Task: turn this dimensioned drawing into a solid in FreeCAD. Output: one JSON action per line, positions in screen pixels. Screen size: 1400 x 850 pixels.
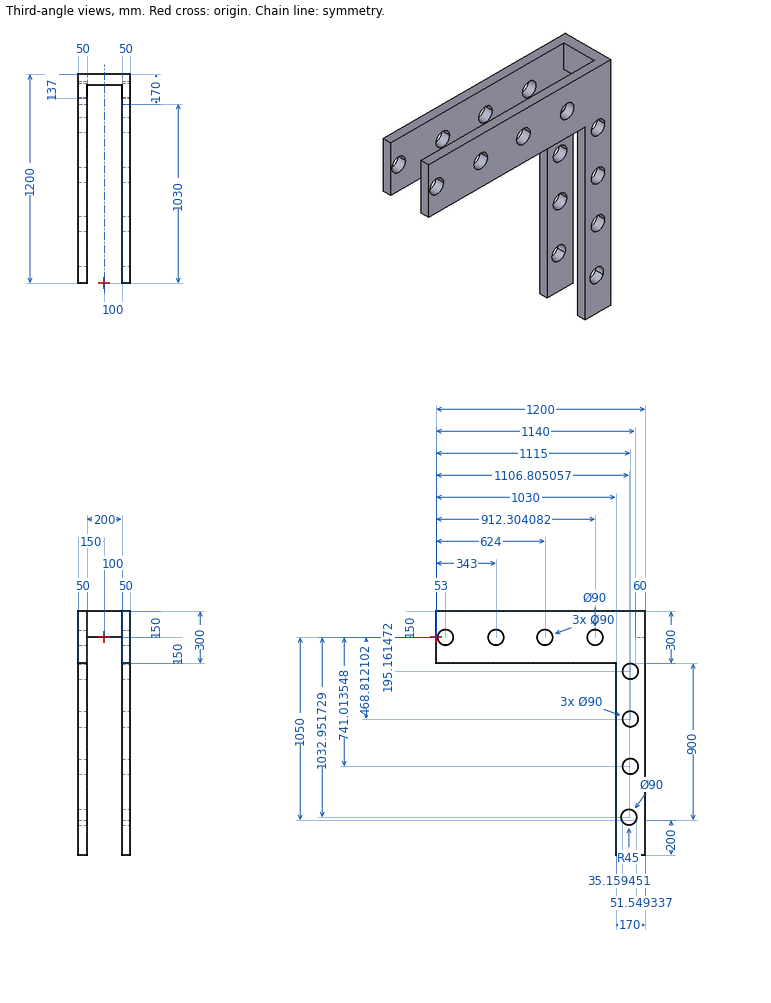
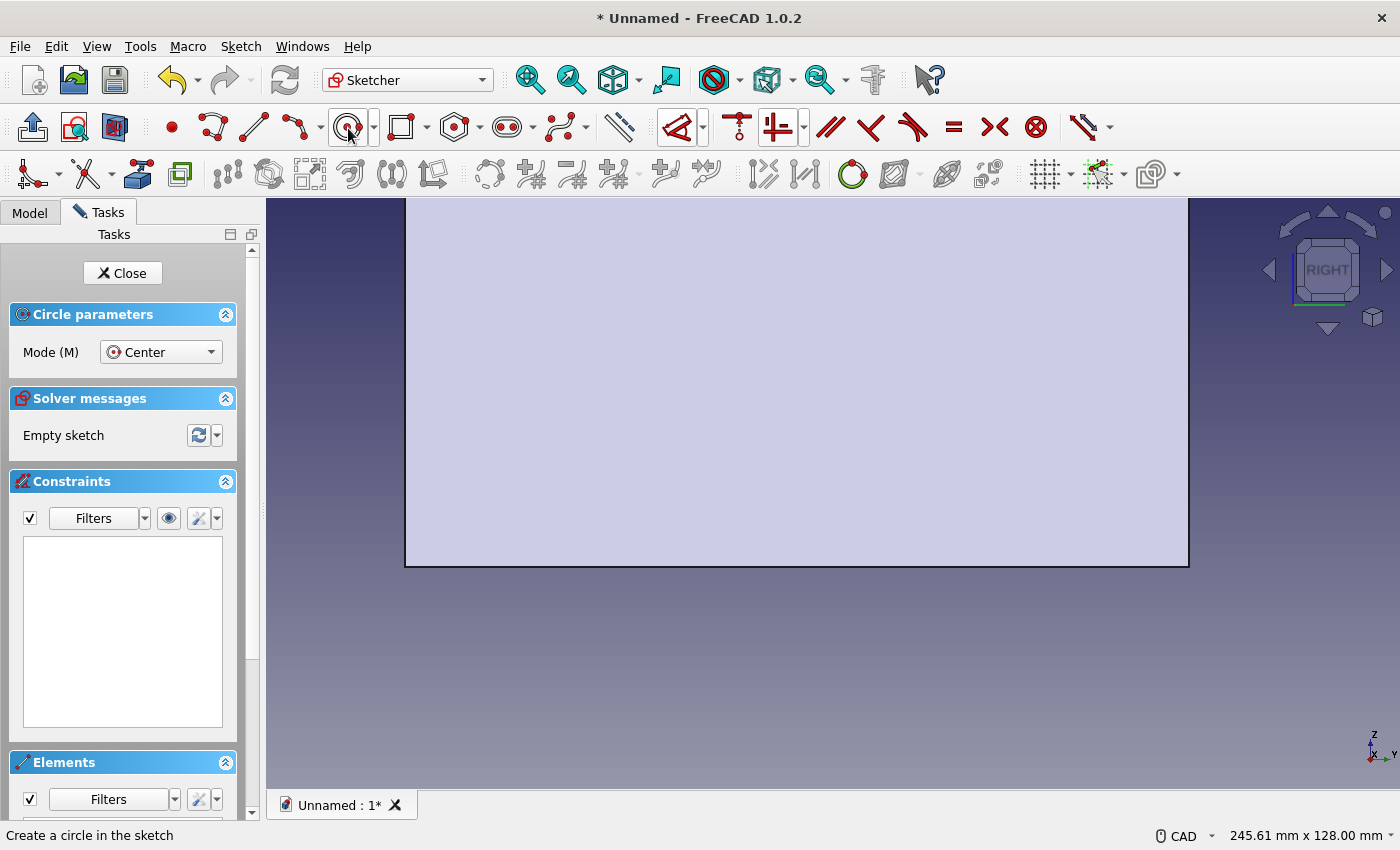
{"action": "left_click", "coordinate": [759, 488]}
{"action": "left_click", "coordinate": [906, 341]}
{"action": "key", "text": "Escape"}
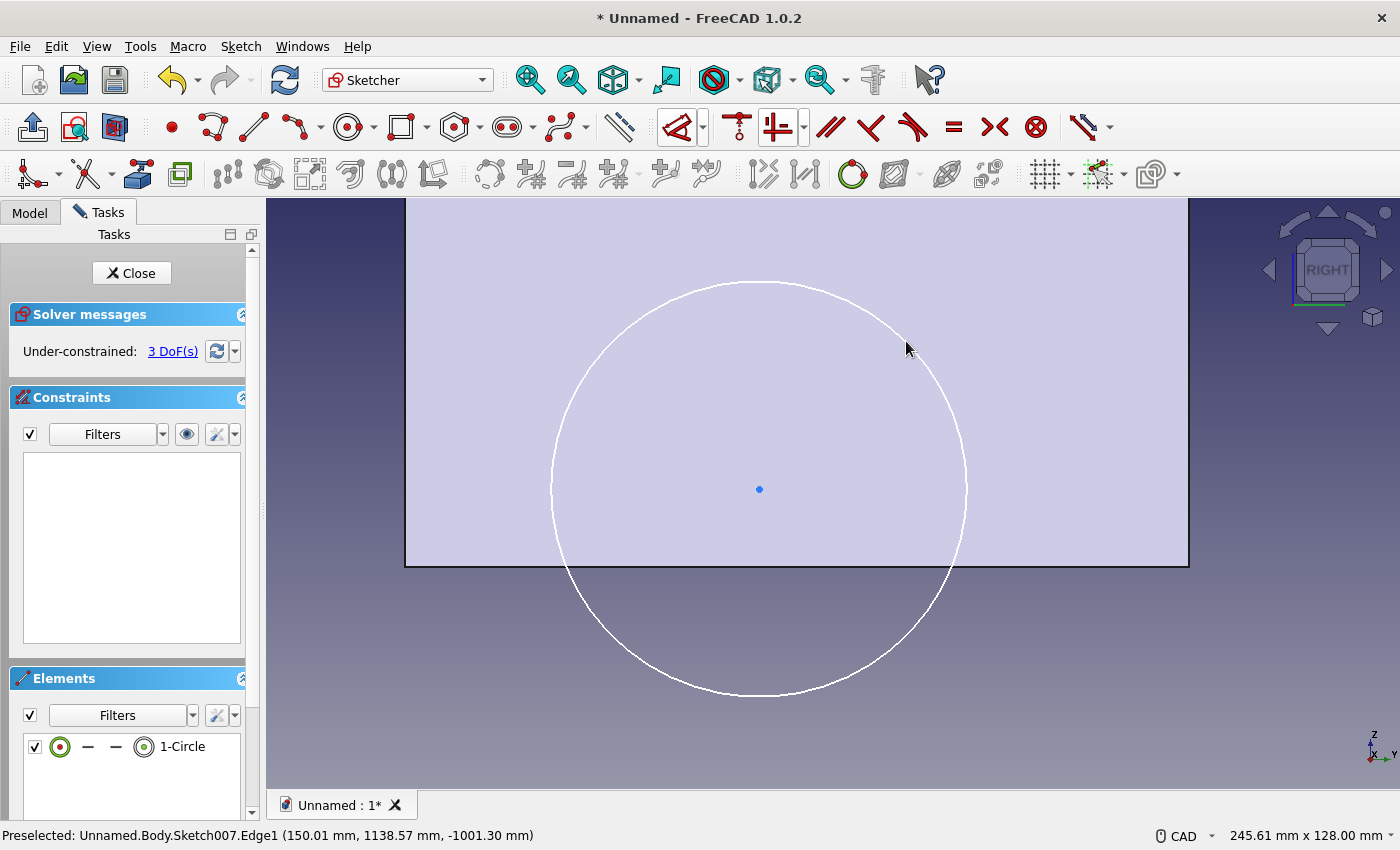
{"action": "left_click", "coordinate": [906, 342]}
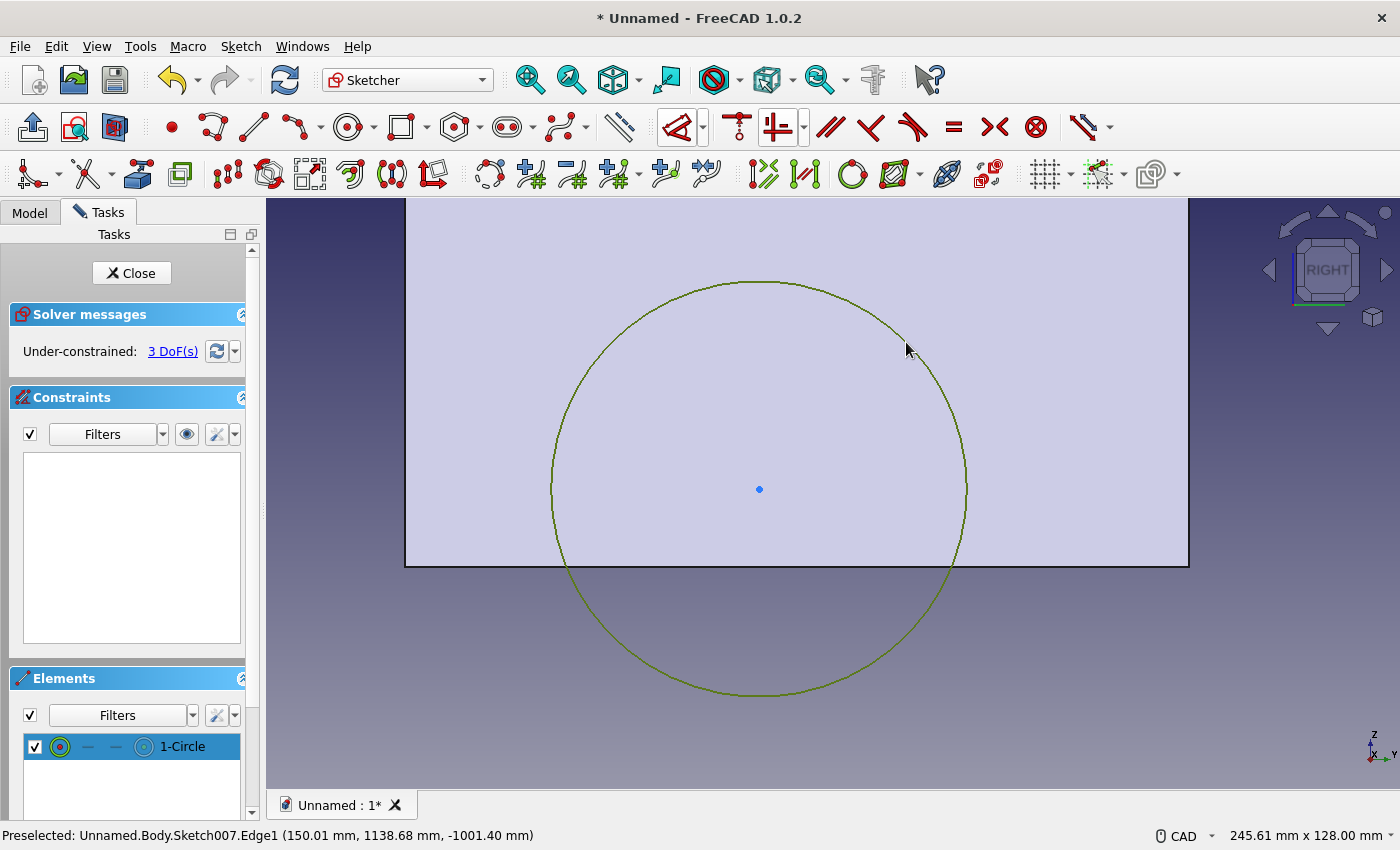
{"action": "key", "text": "k o"}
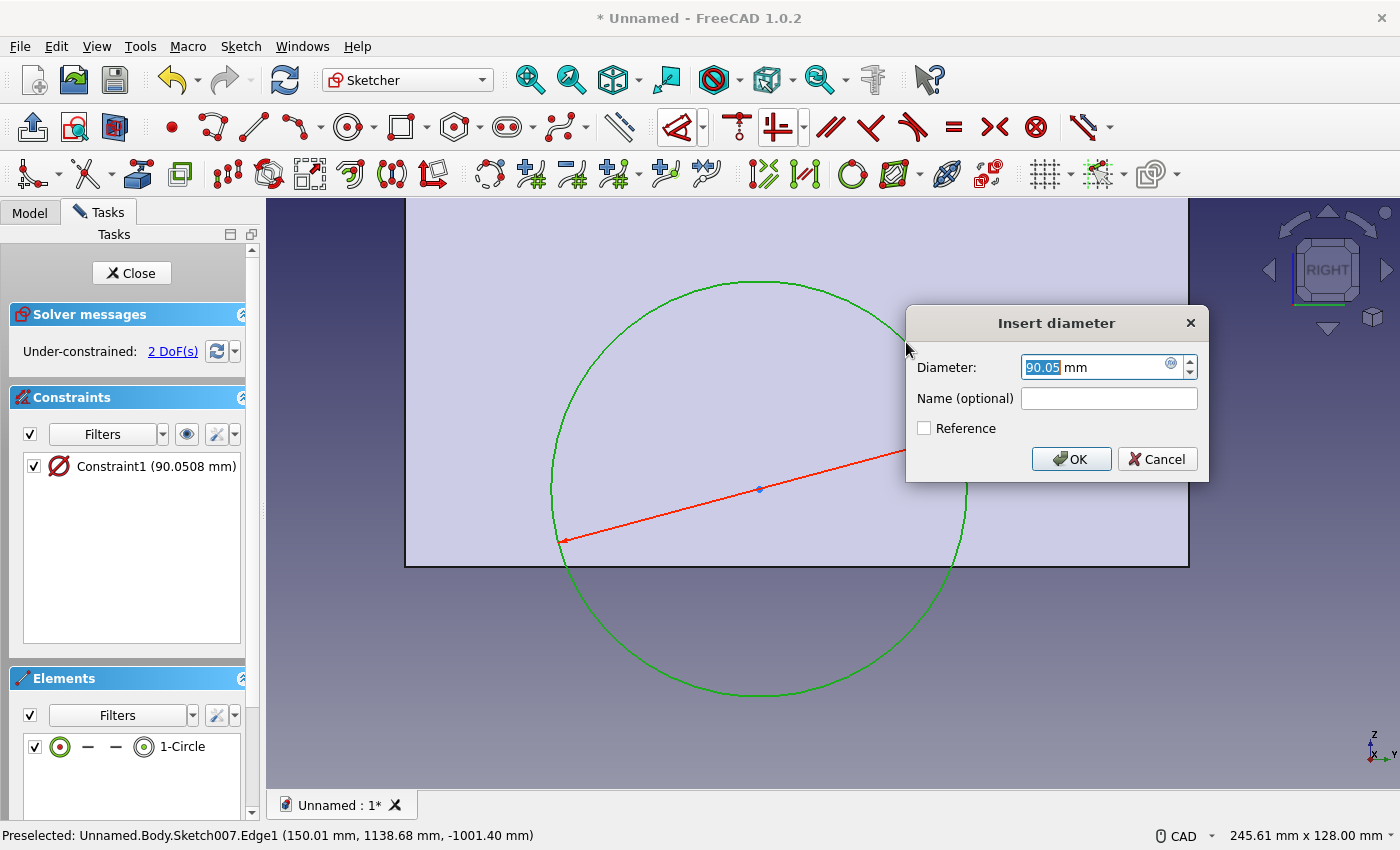
{"action": "type", "text": "90"}
{"action": "key", "text": "Return"}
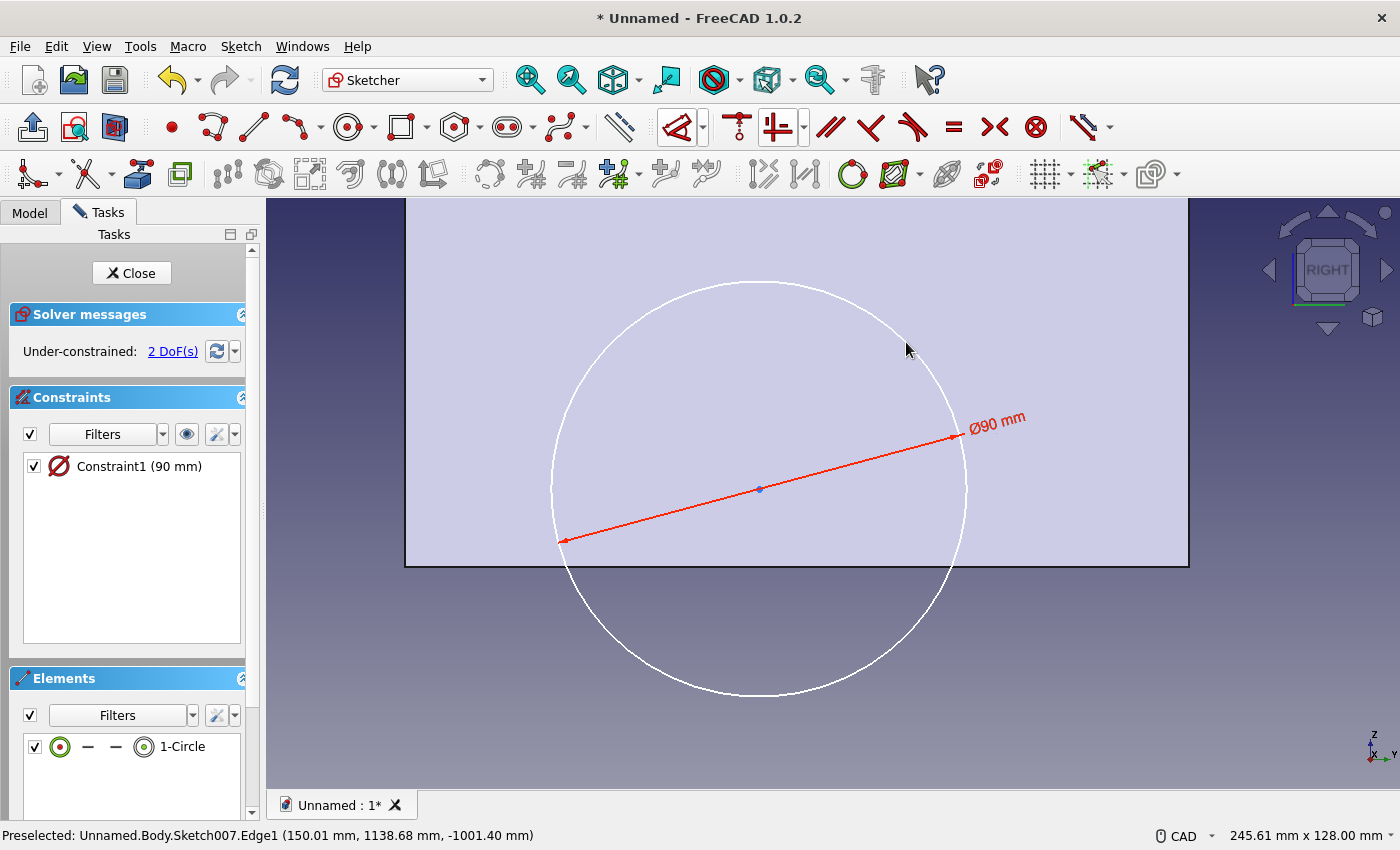
{"action": "left_click", "coordinate": [759, 489]}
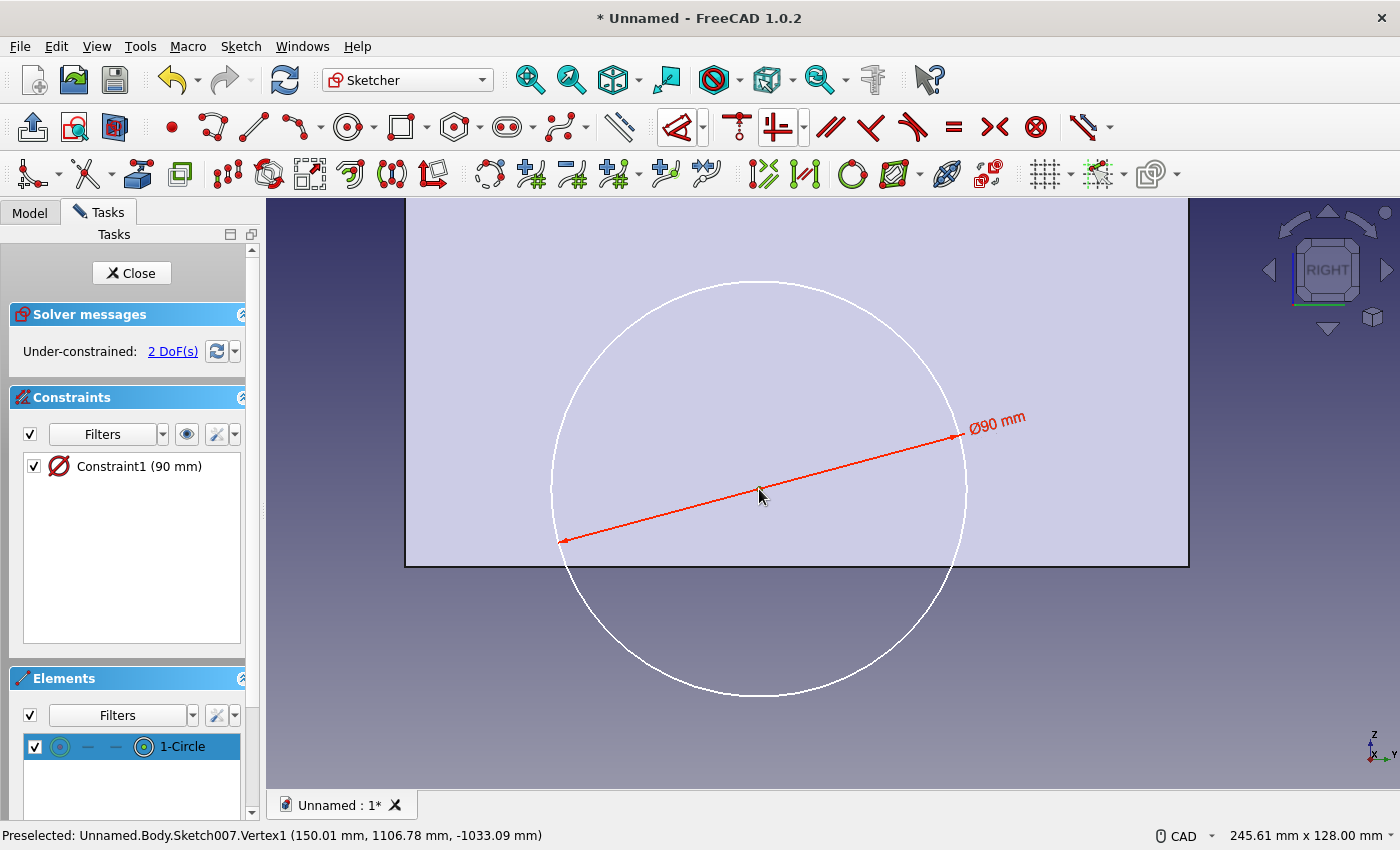
{"action": "left_click", "coordinate": [702, 128]}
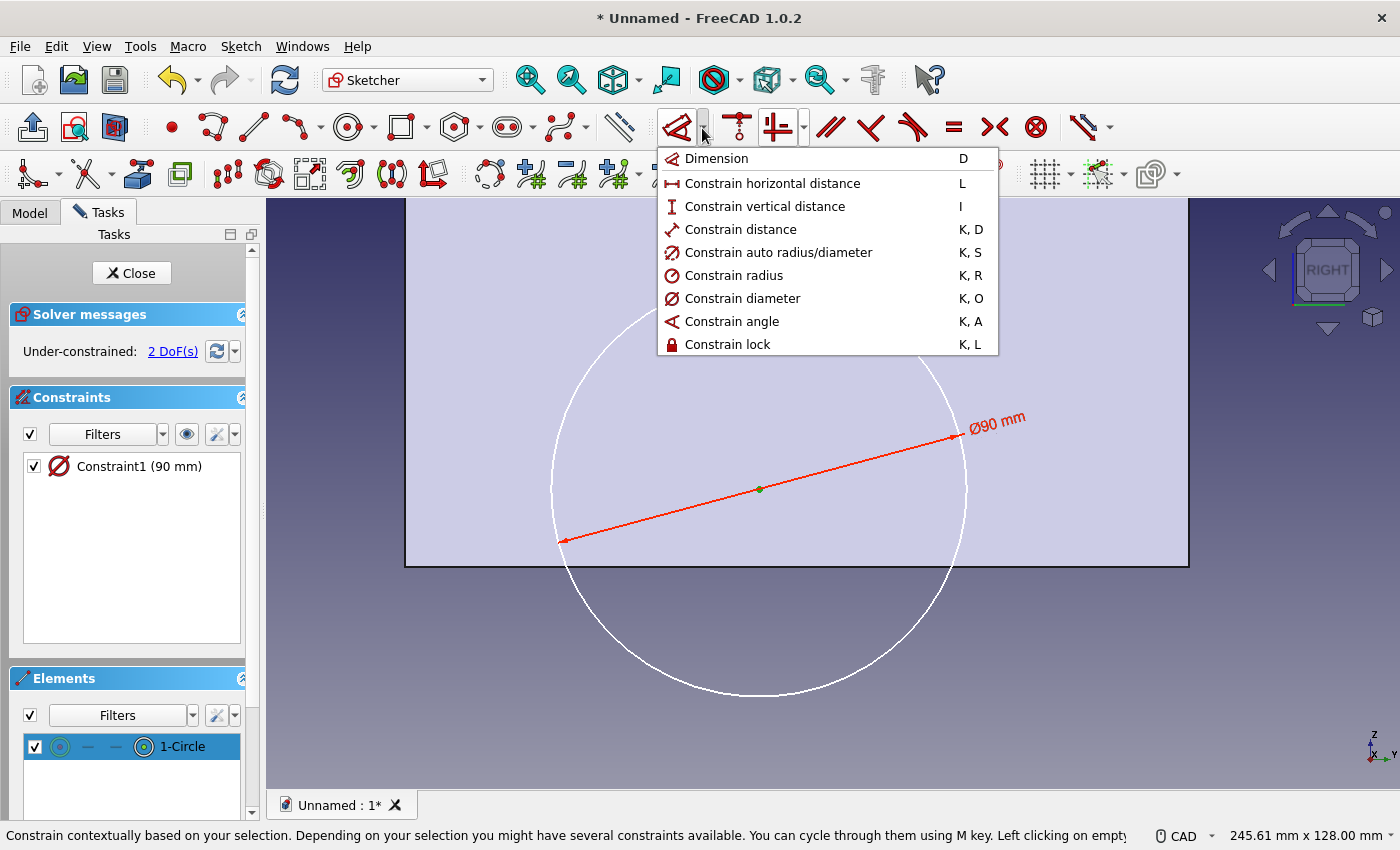
{"action": "left_click", "coordinate": [828, 184]}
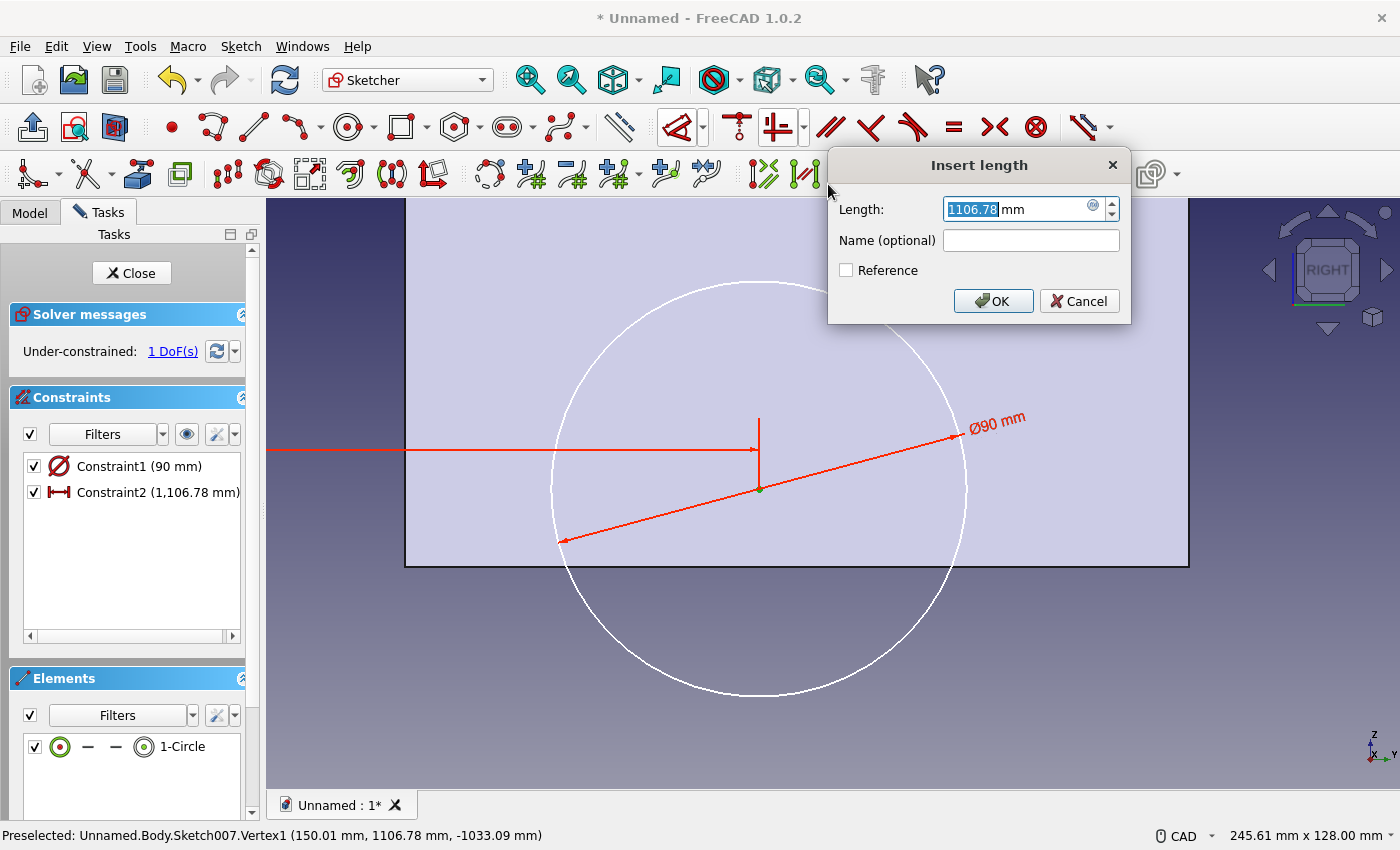
{"action": "type", "text": "1106.805057"}
{"action": "key", "text": "Return"}